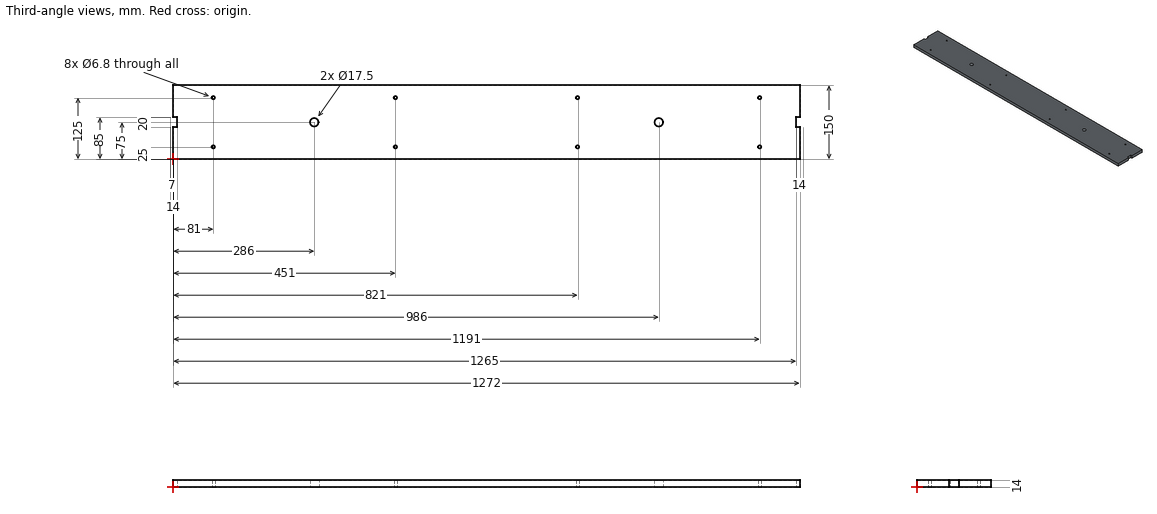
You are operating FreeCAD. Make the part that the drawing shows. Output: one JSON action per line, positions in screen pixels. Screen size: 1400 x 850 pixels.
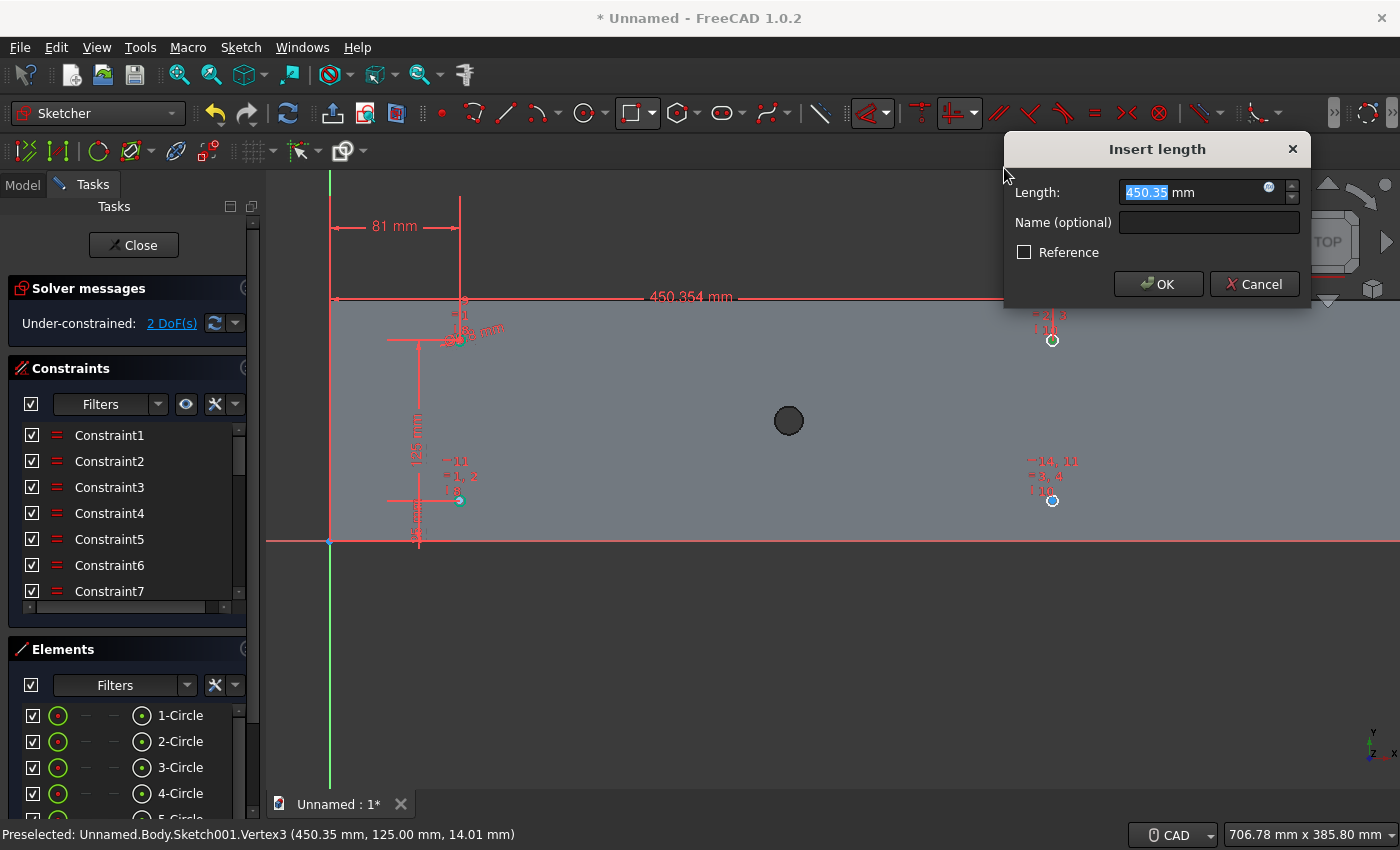
{"action": "type", "text": "451"}
{"action": "key", "text": "Return"}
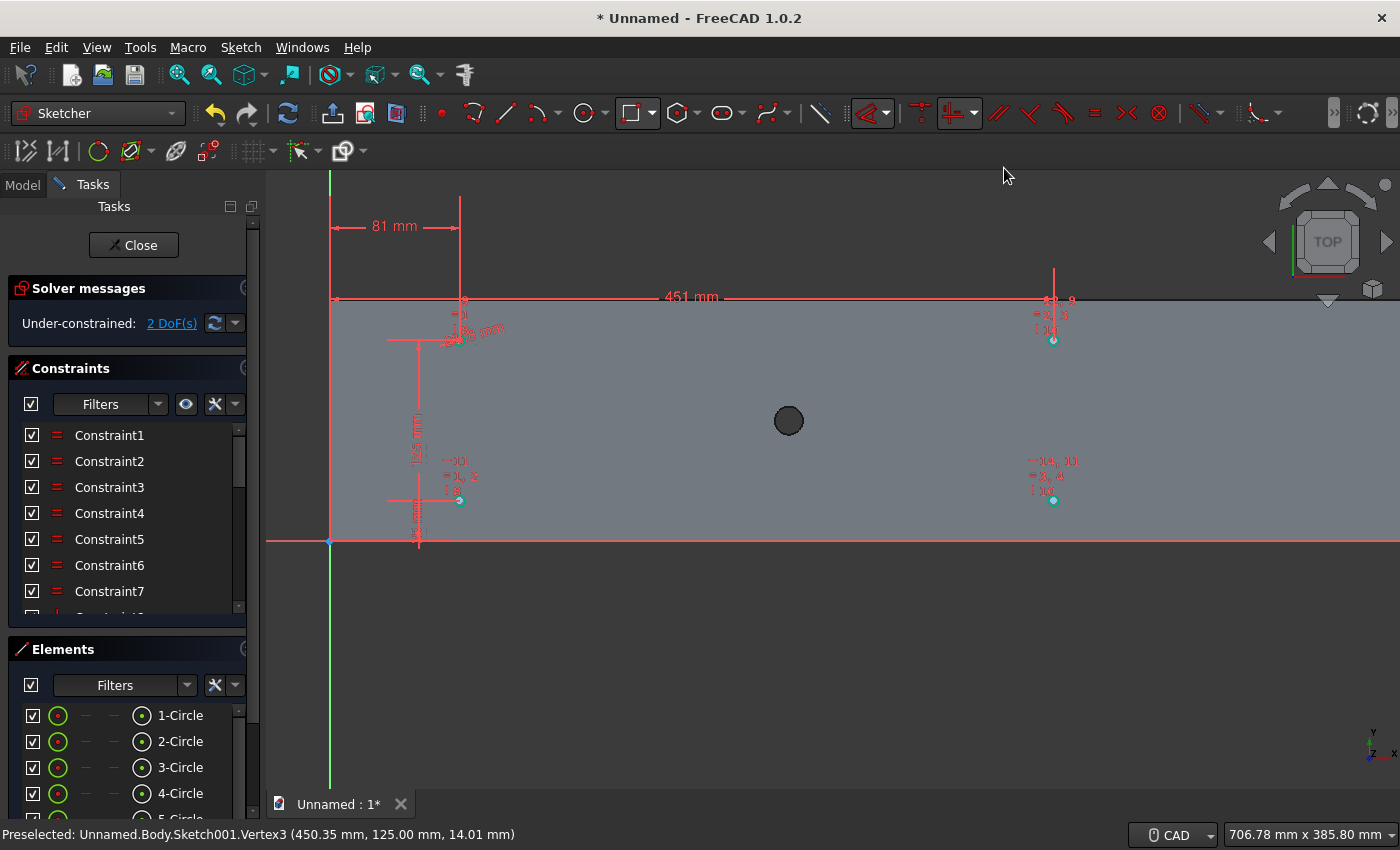
{"action": "scroll", "coordinate": [460, 504], "scroll_direction": "down", "scroll_amount": 5}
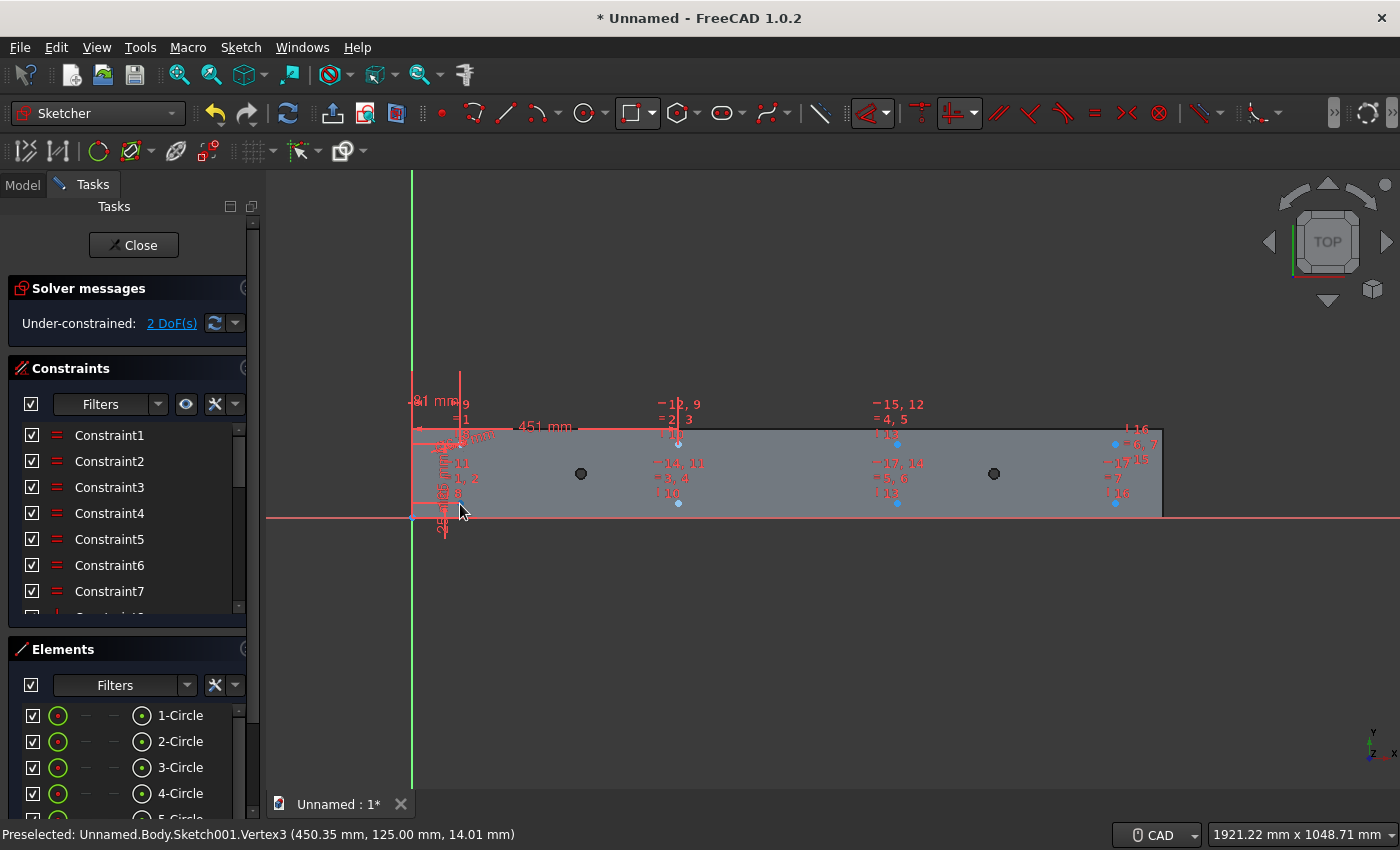
{"action": "left_click", "coordinate": [897, 444]}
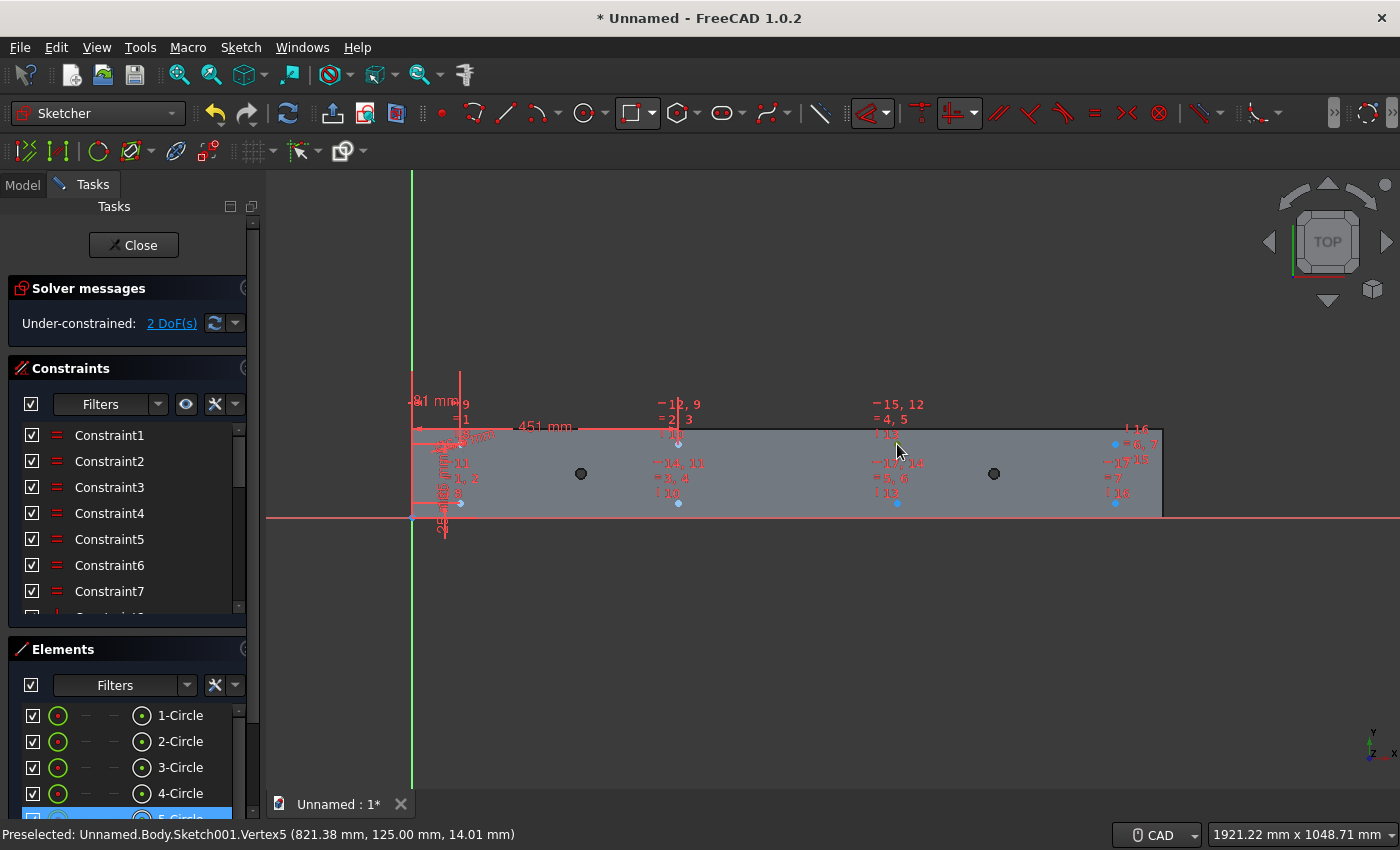
{"action": "key", "text": "l"}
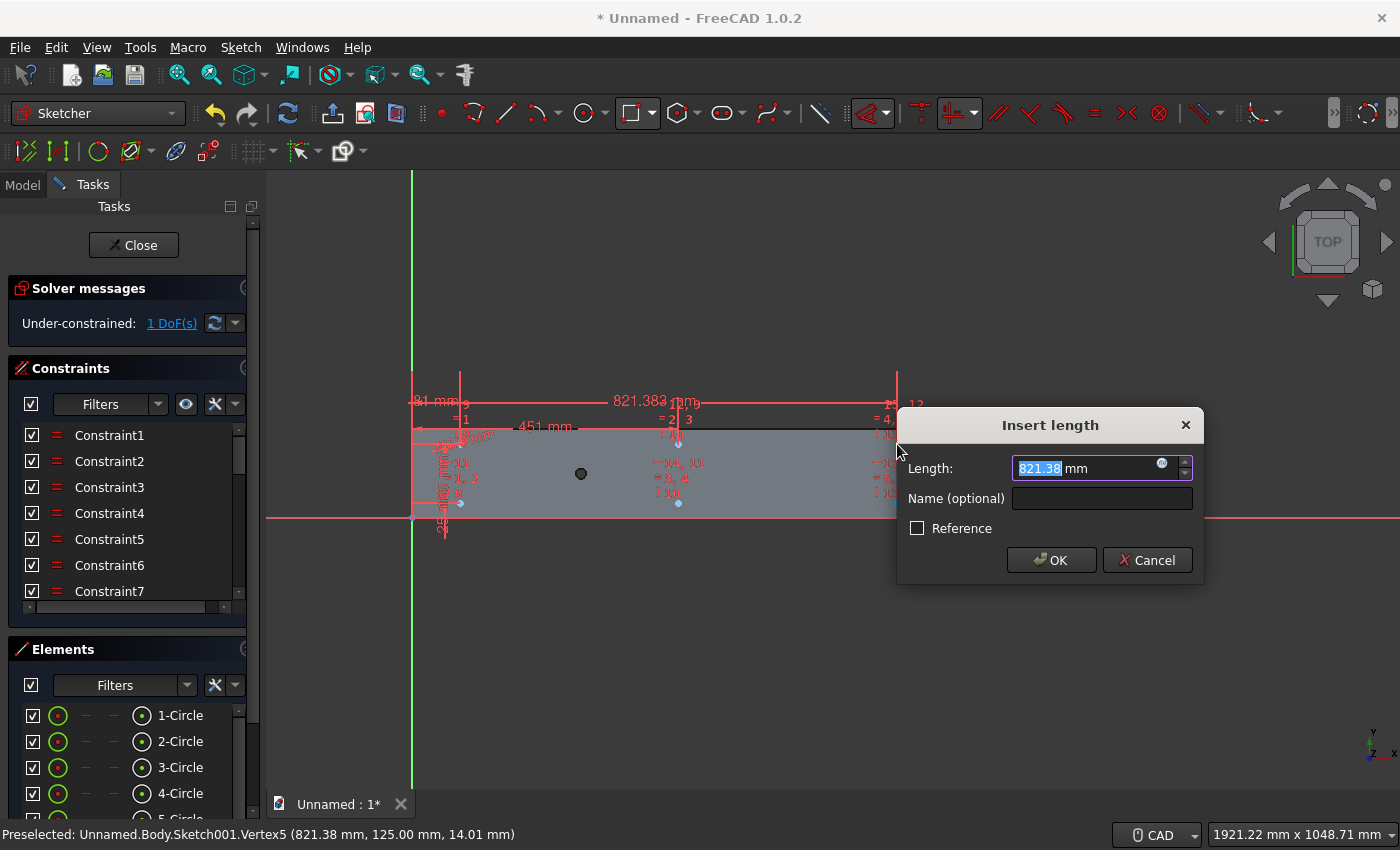
{"action": "type", "text": "821"}
{"action": "key", "text": "Return"}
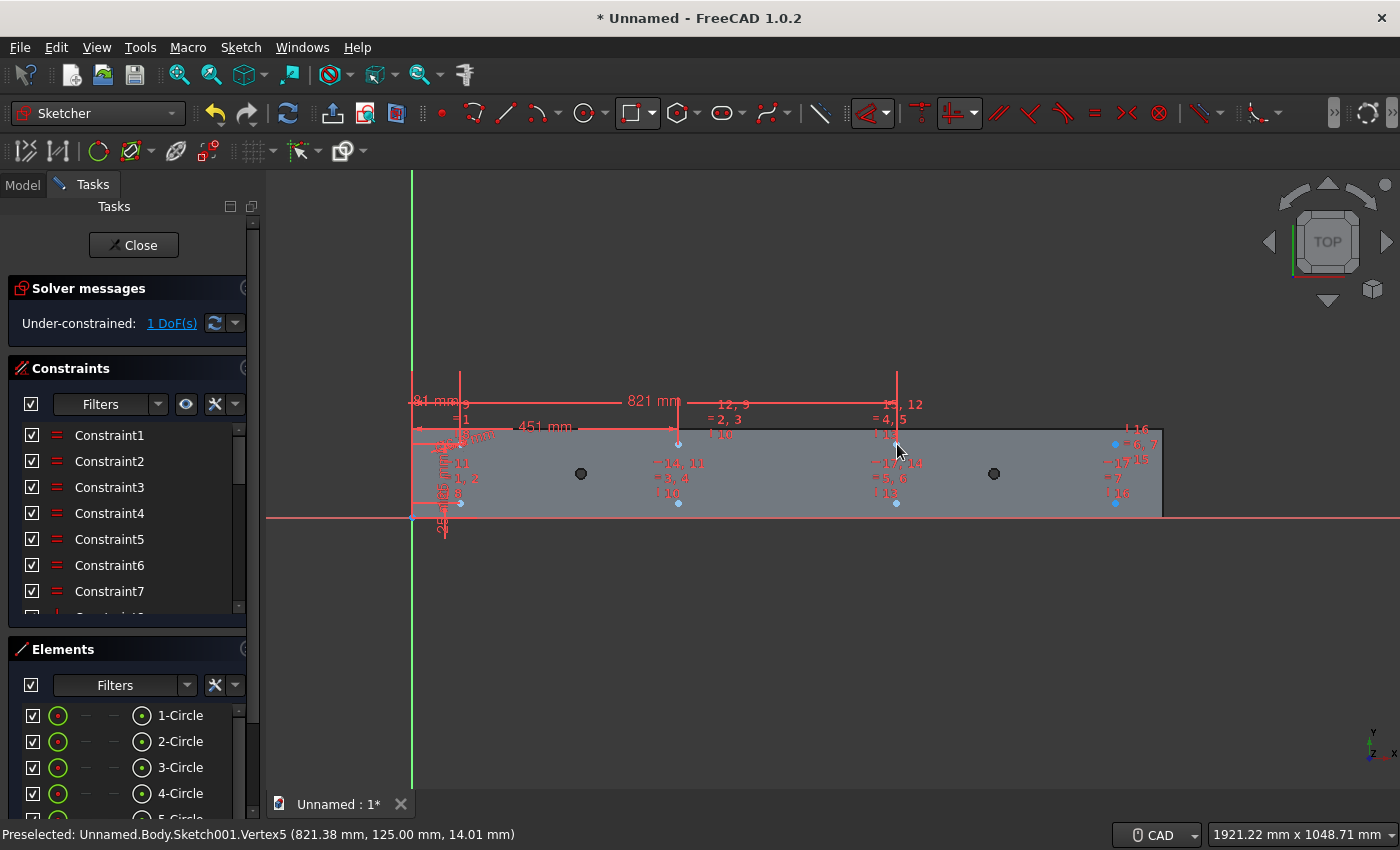
{"action": "left_click", "coordinate": [1115, 444]}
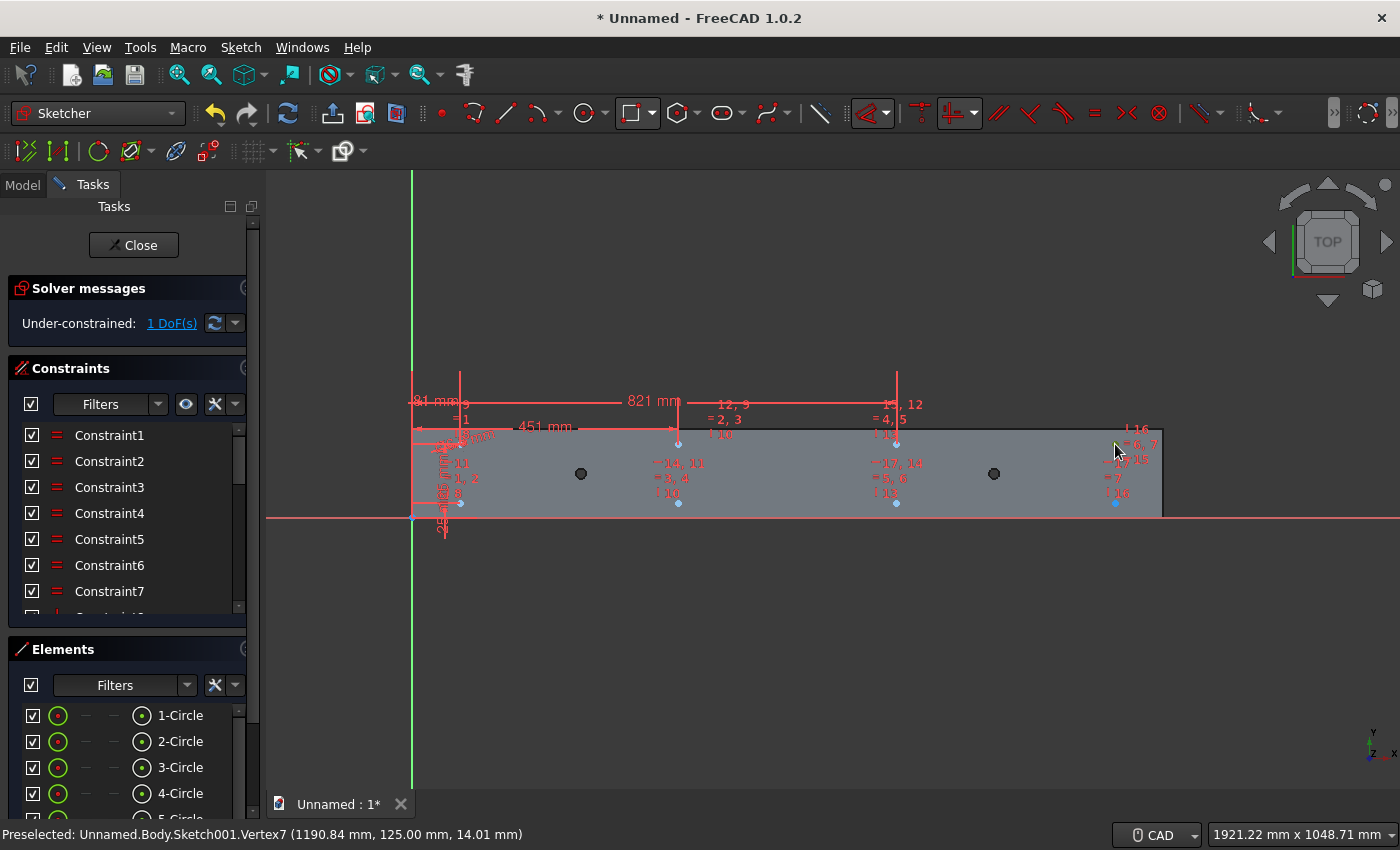
{"action": "left_click", "coordinate": [888, 114]}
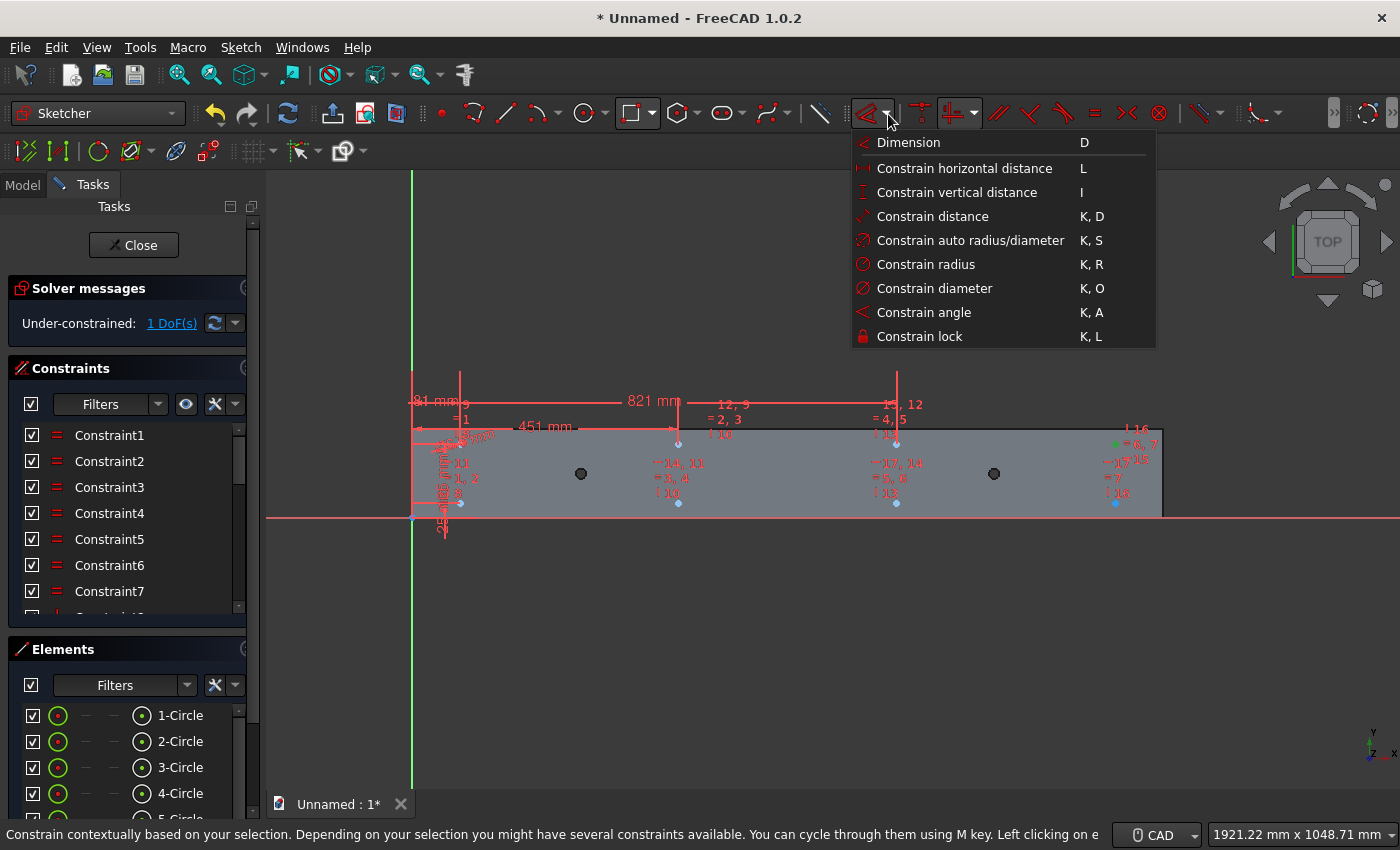
{"action": "left_click", "coordinate": [1004, 168]}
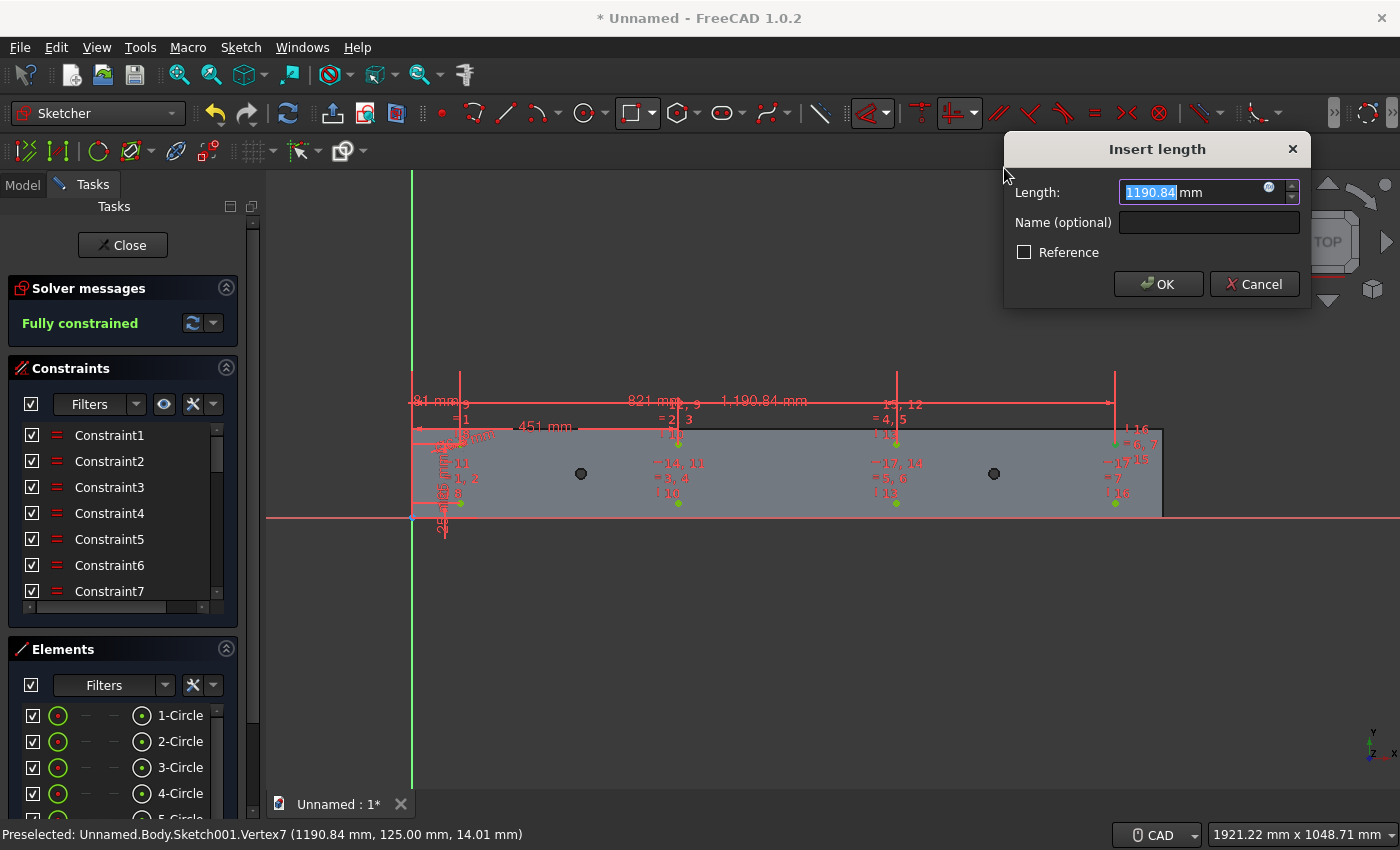
{"action": "type", "text": "1191"}
{"action": "key", "text": "Return"}